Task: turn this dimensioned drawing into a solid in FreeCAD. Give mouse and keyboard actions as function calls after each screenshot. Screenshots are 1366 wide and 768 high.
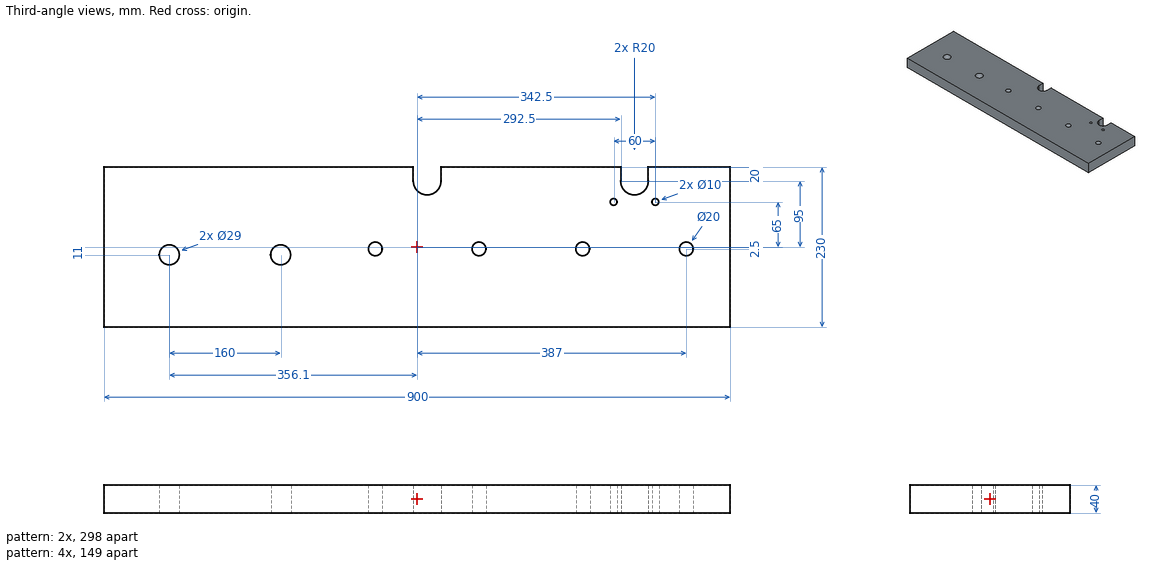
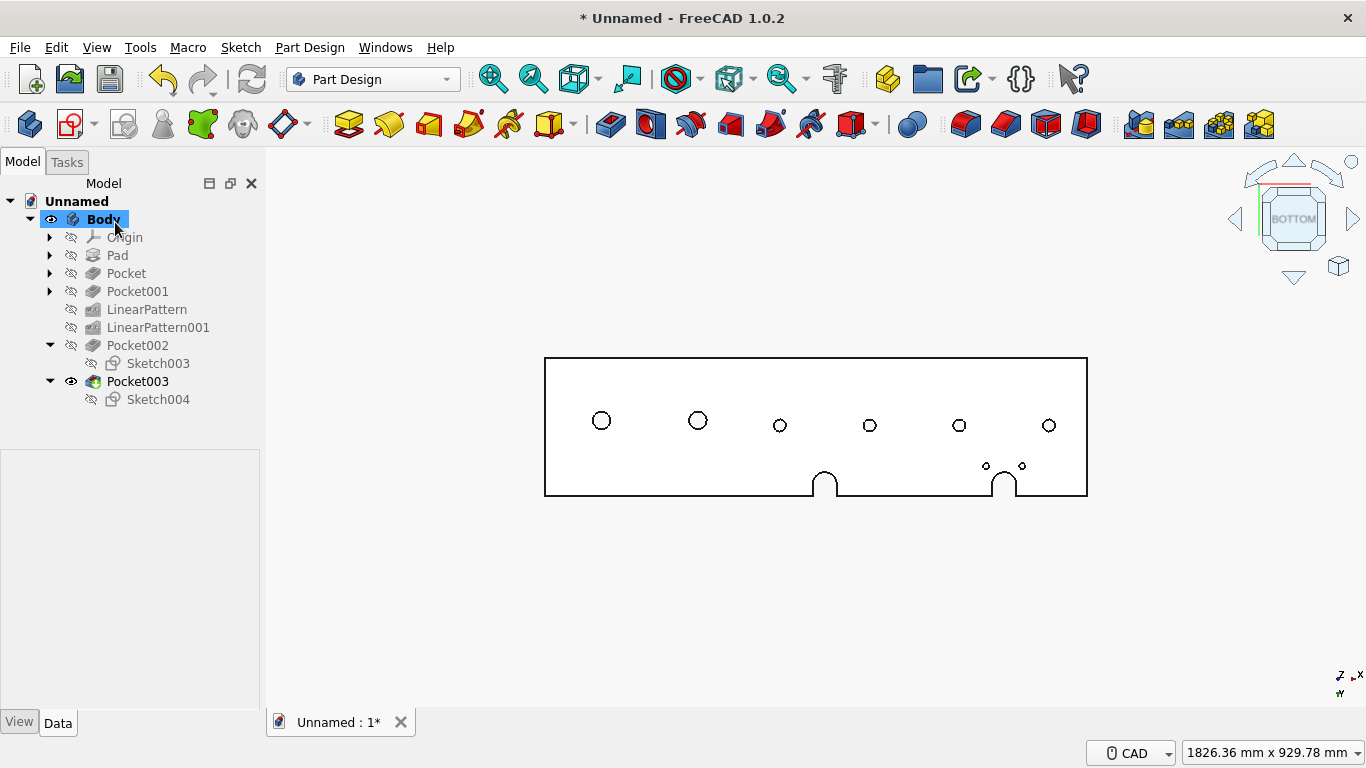
key(0)